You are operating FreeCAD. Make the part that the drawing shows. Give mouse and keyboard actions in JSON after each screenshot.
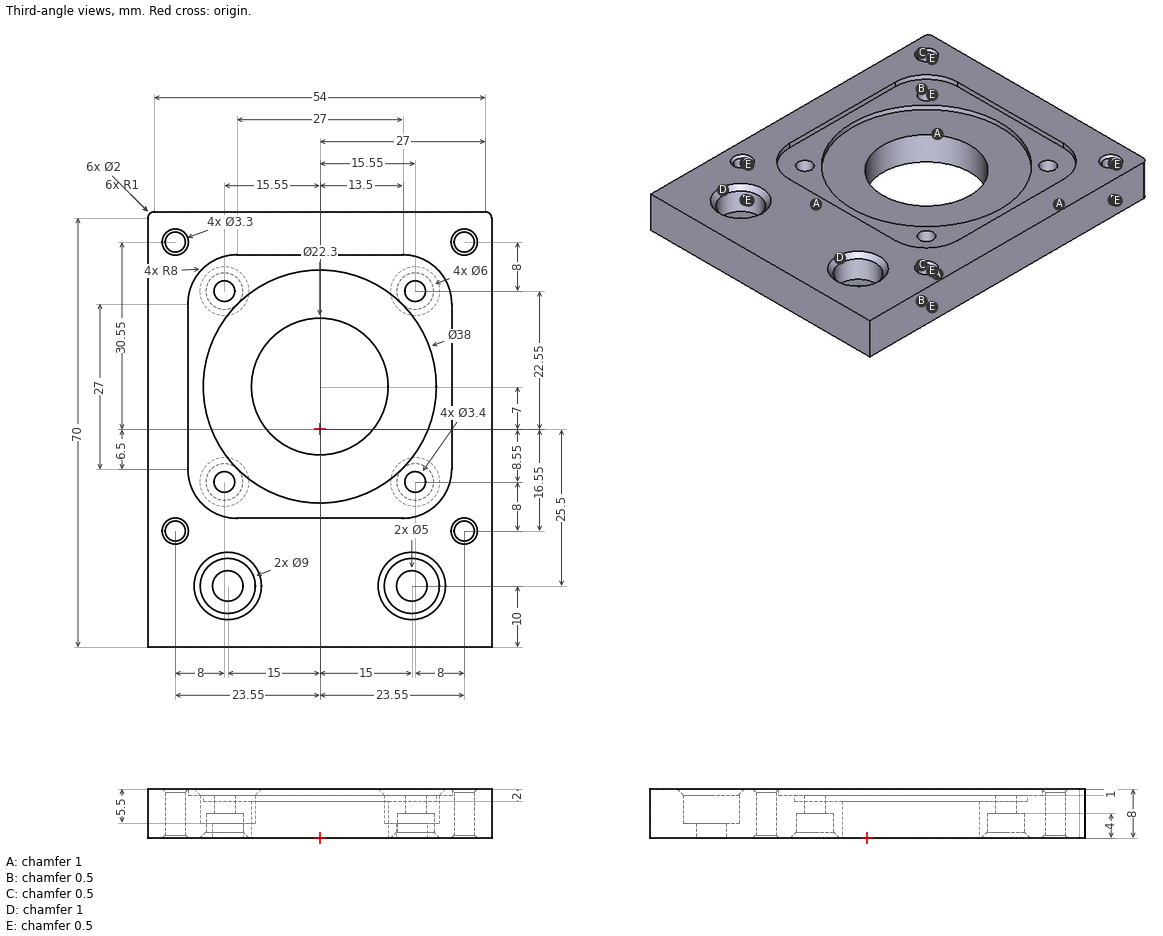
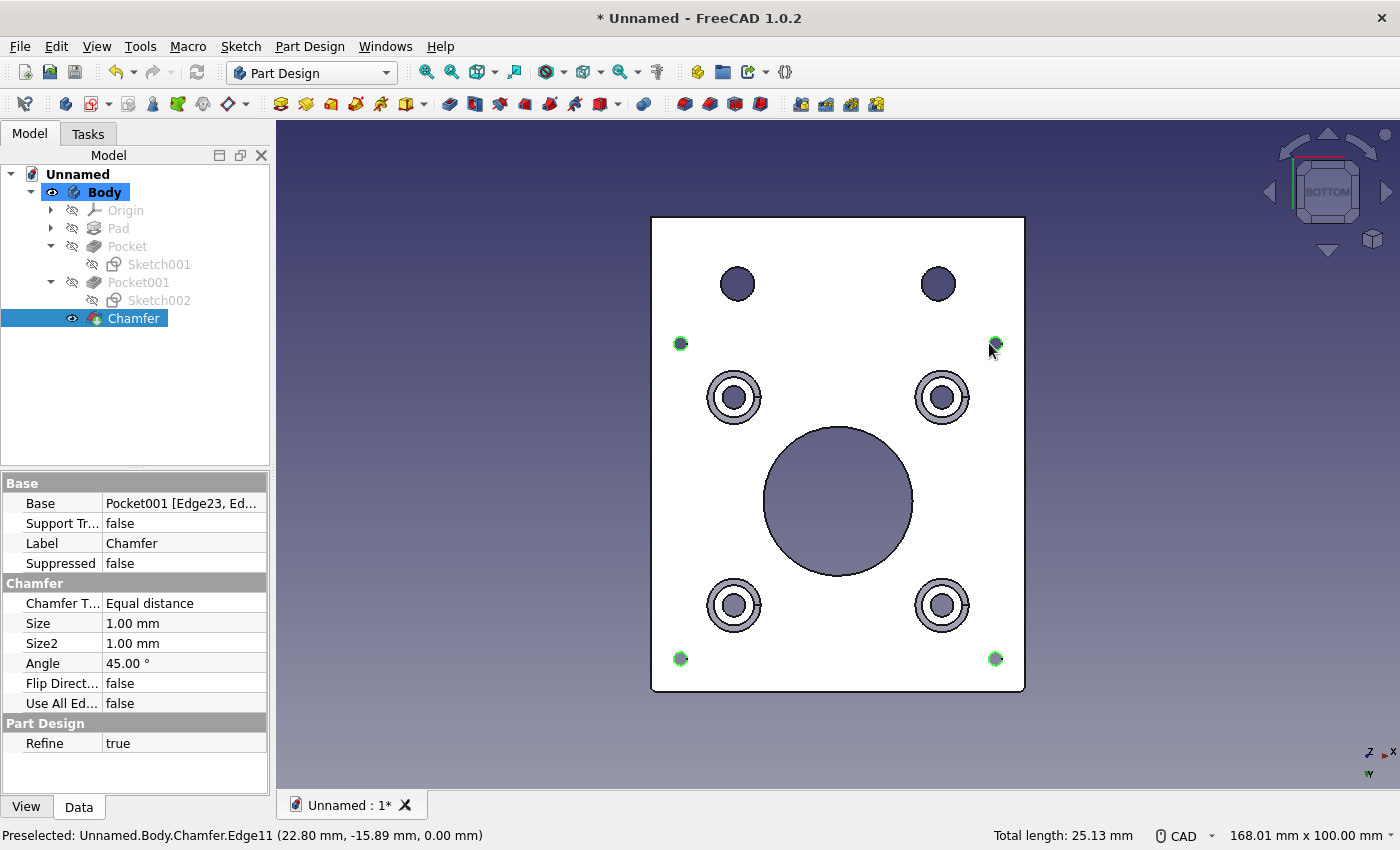
{"action": "left_click", "coordinate": [710, 104]}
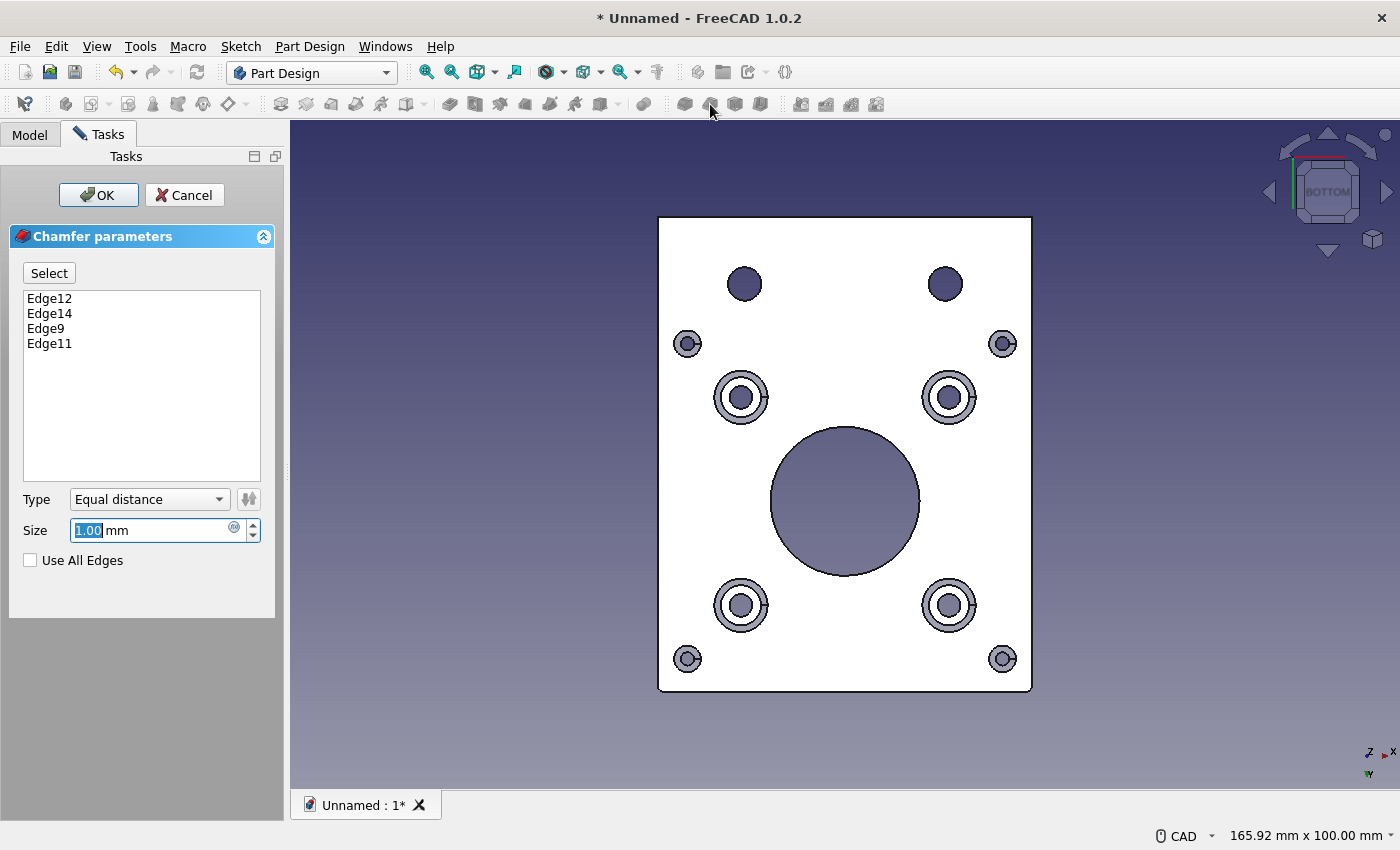
{"action": "type", "text": "0.5"}
{"action": "key", "text": "Tab"}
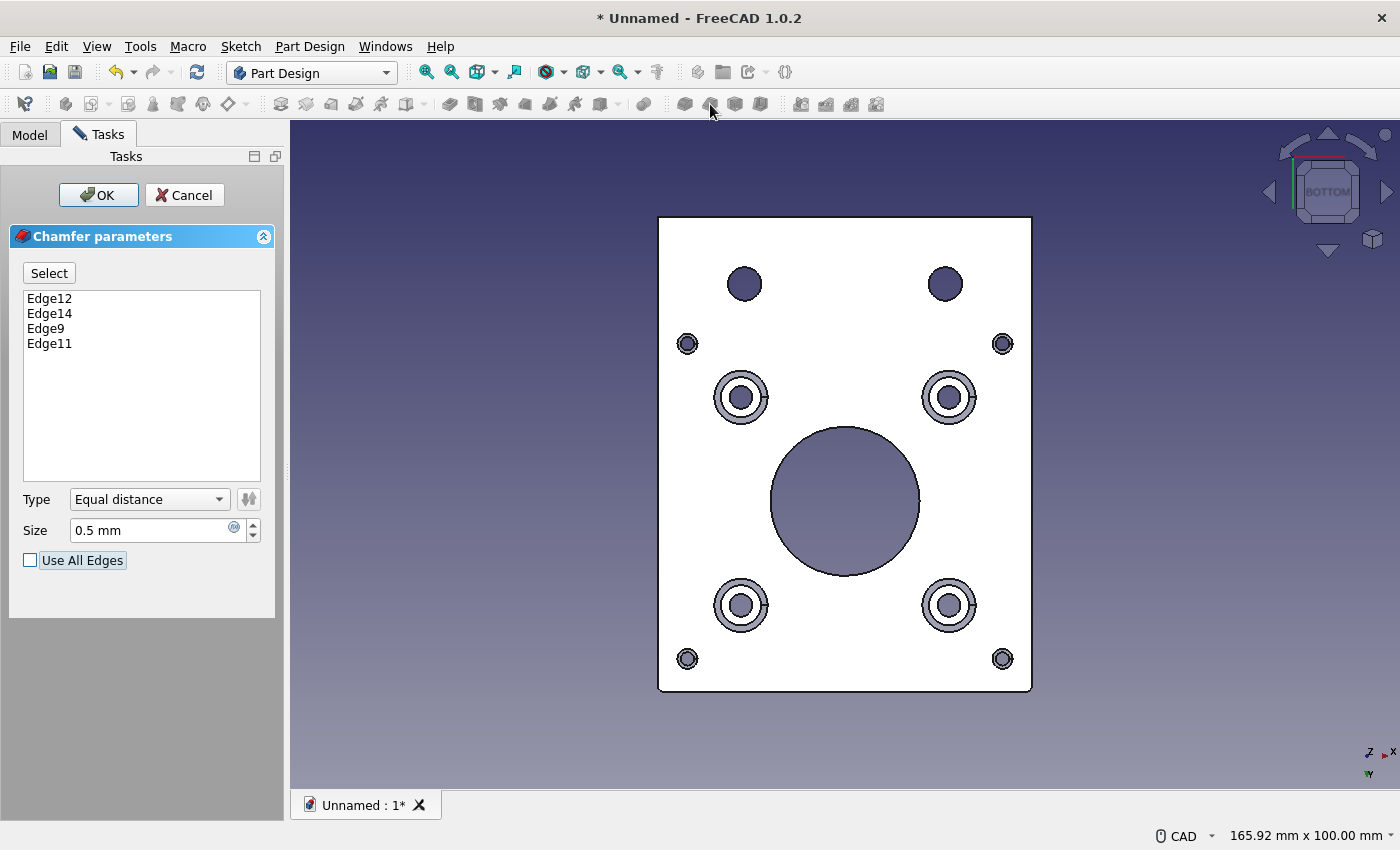
{"action": "left_click", "coordinate": [99, 195]}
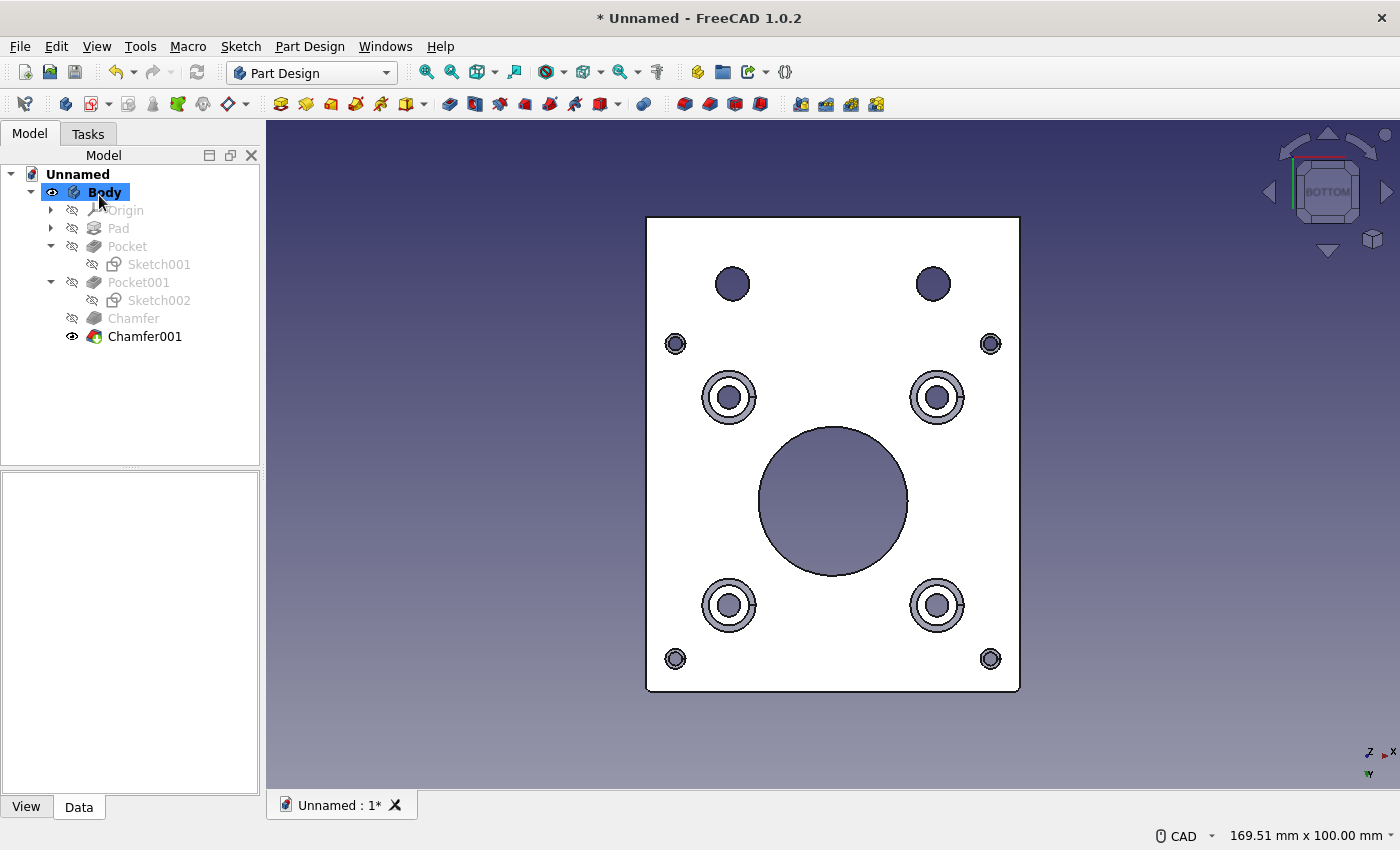
{"action": "key", "text": "0"}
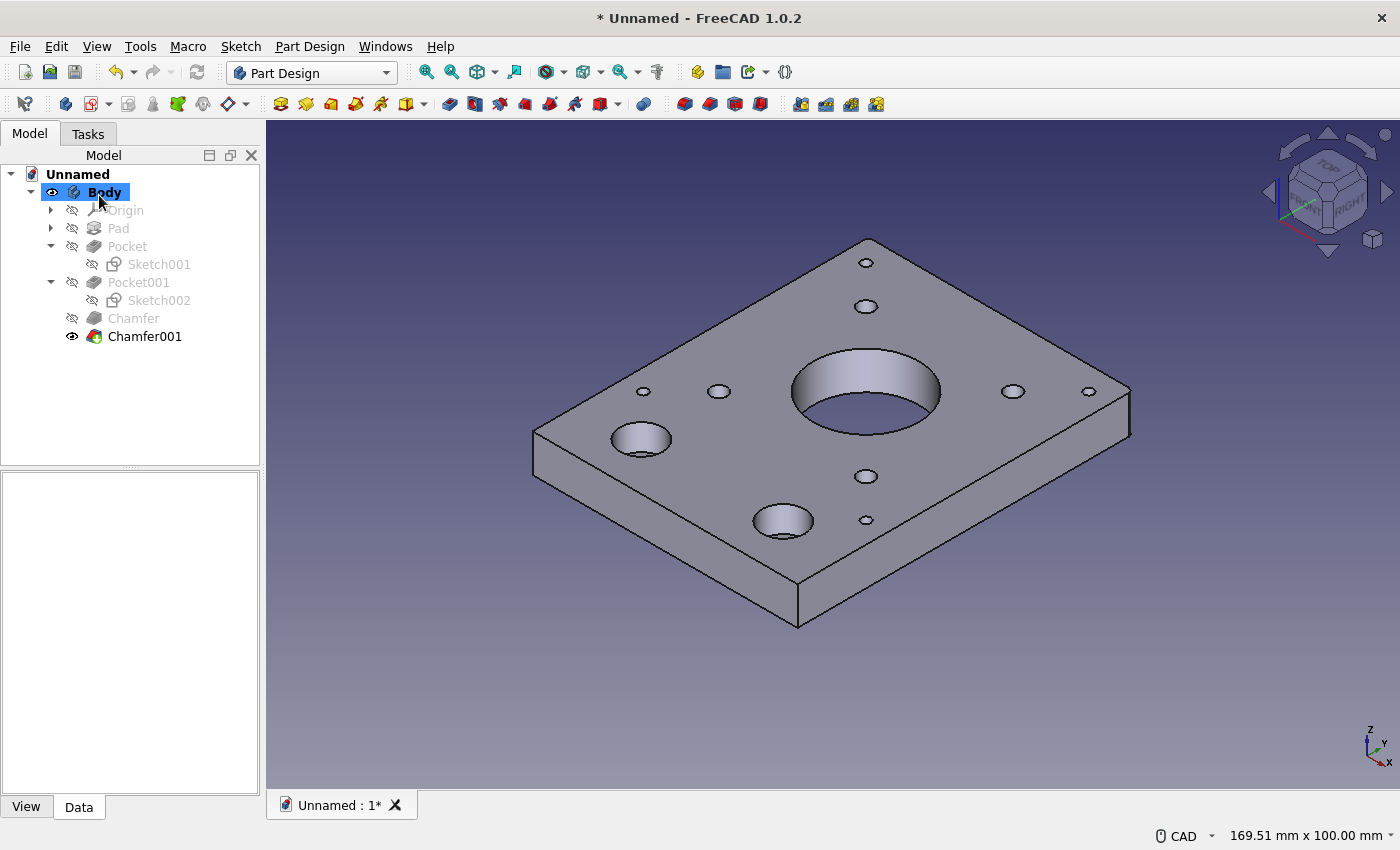
{"action": "left_click", "coordinate": [861, 259]}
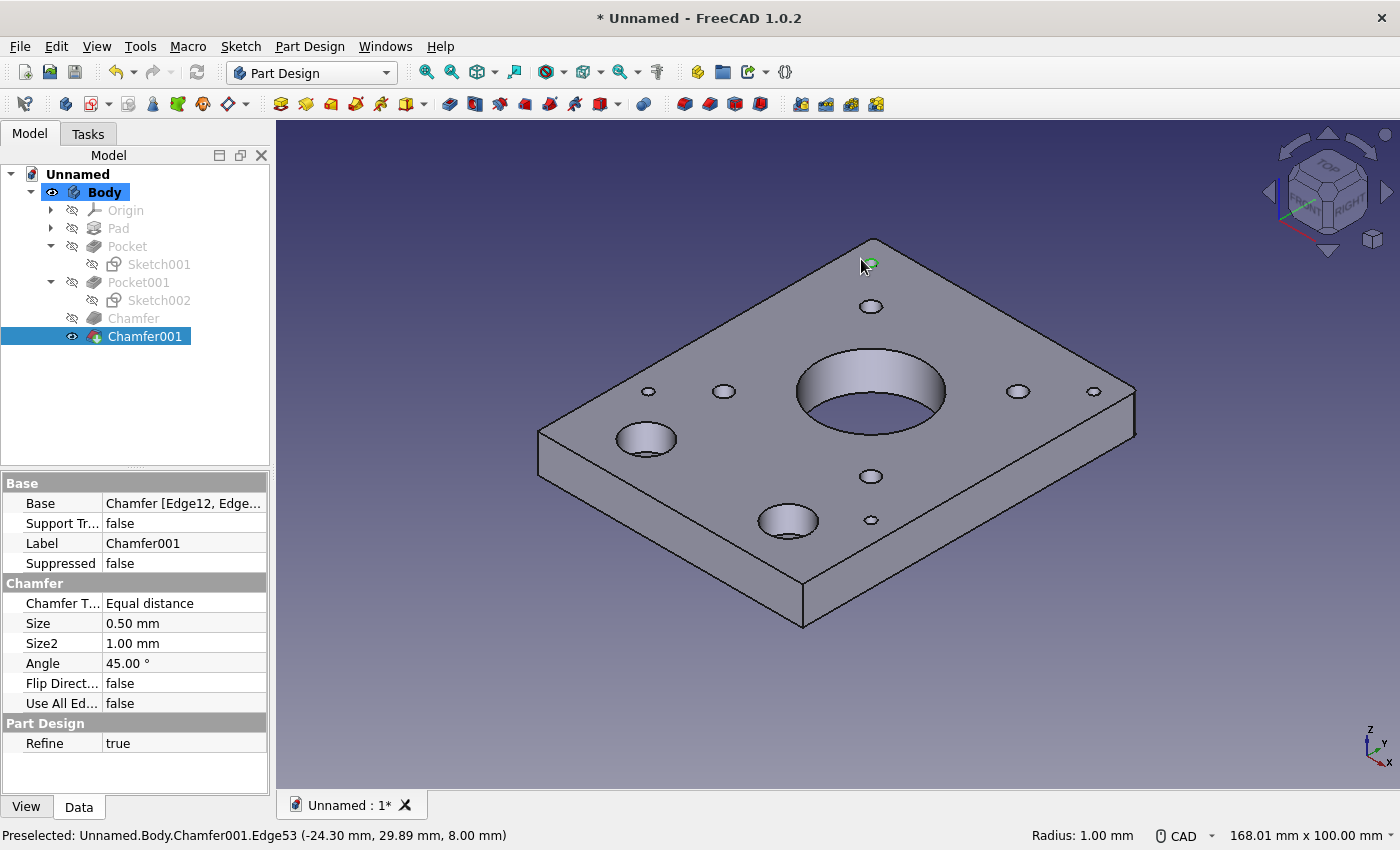
{"action": "left_click", "coordinate": [1089, 388], "text": "ctrl"}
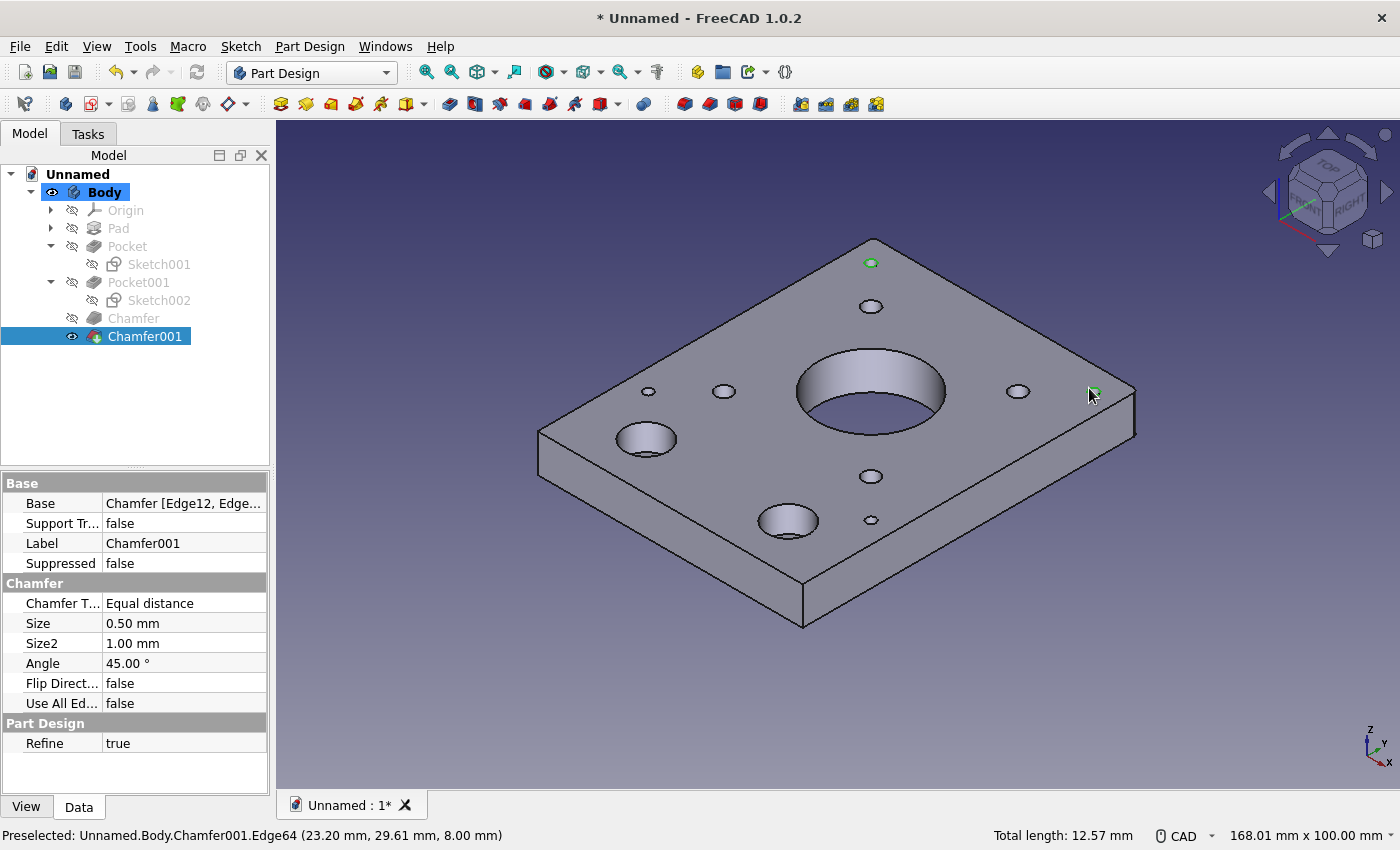
{"action": "left_click", "coordinate": [644, 388], "text": "ctrl"}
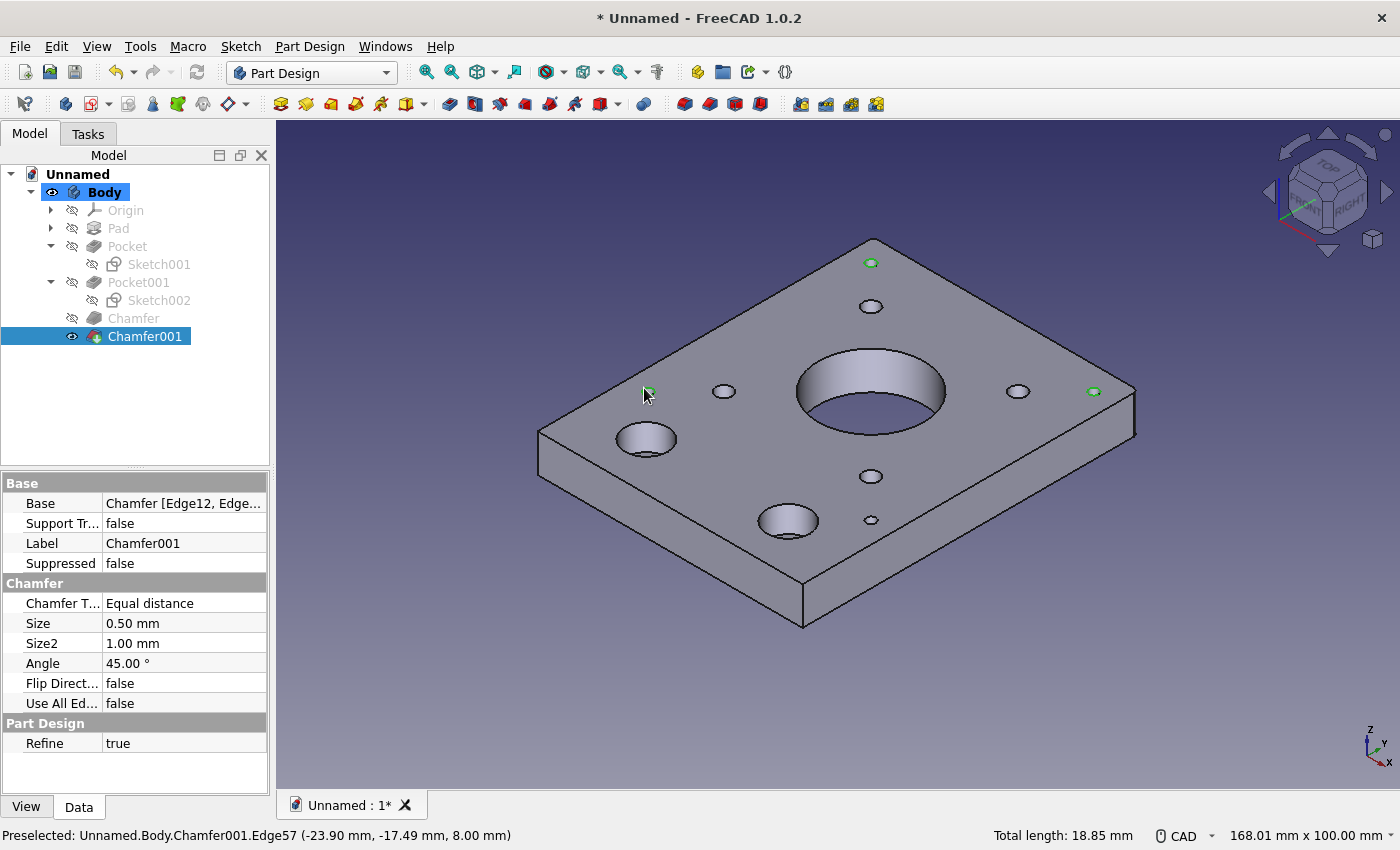
{"action": "left_click", "coordinate": [866, 517], "text": "ctrl"}